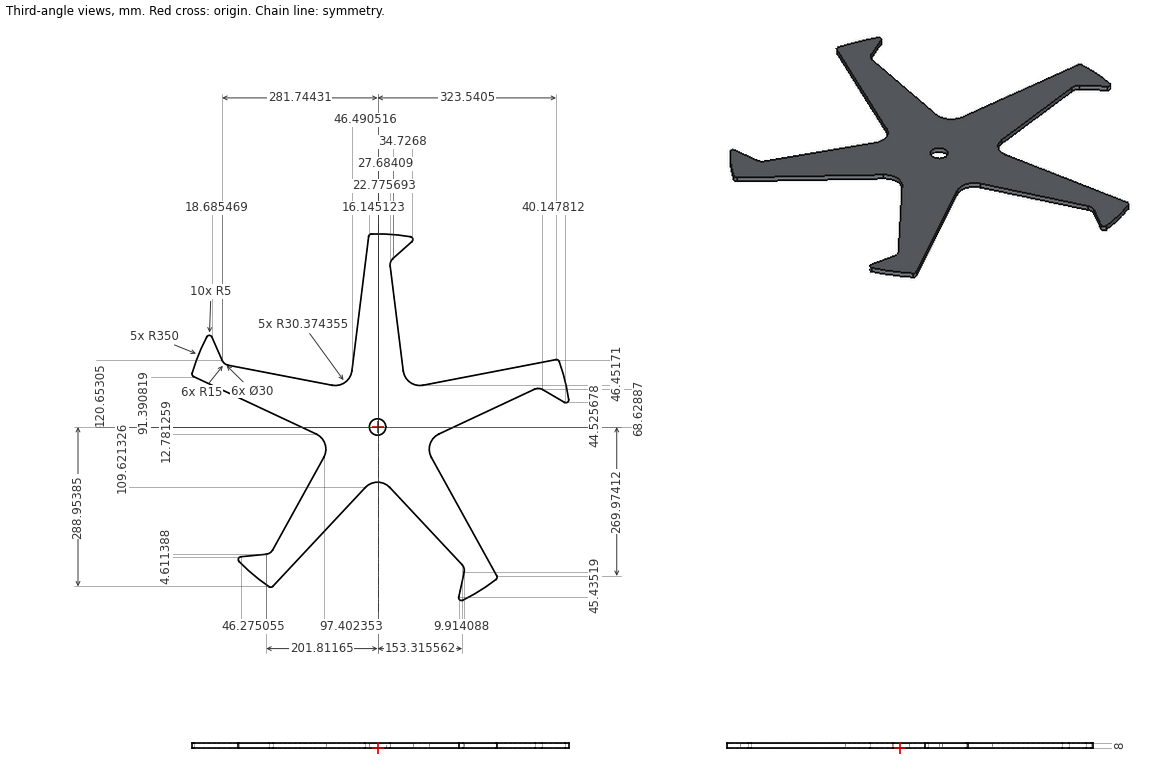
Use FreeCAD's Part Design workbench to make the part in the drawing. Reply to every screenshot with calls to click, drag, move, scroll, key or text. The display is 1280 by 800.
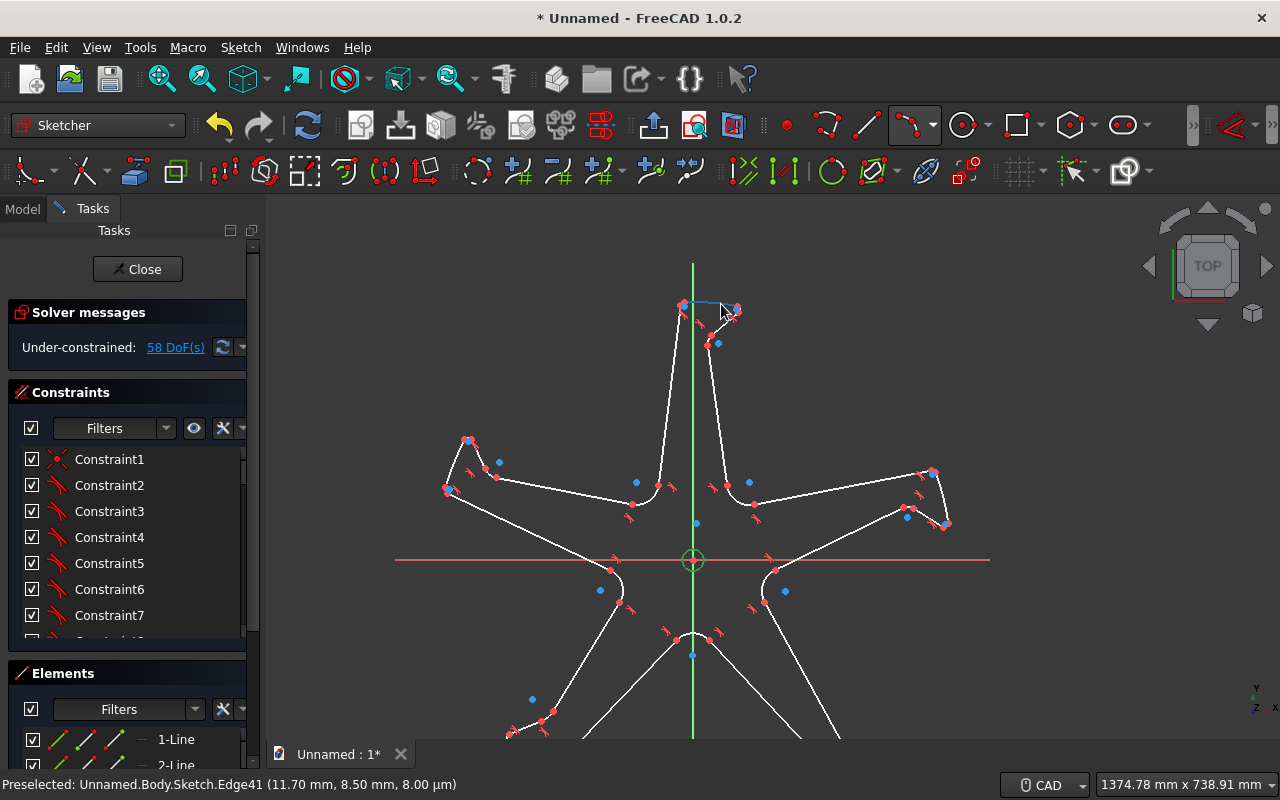
click(722, 304)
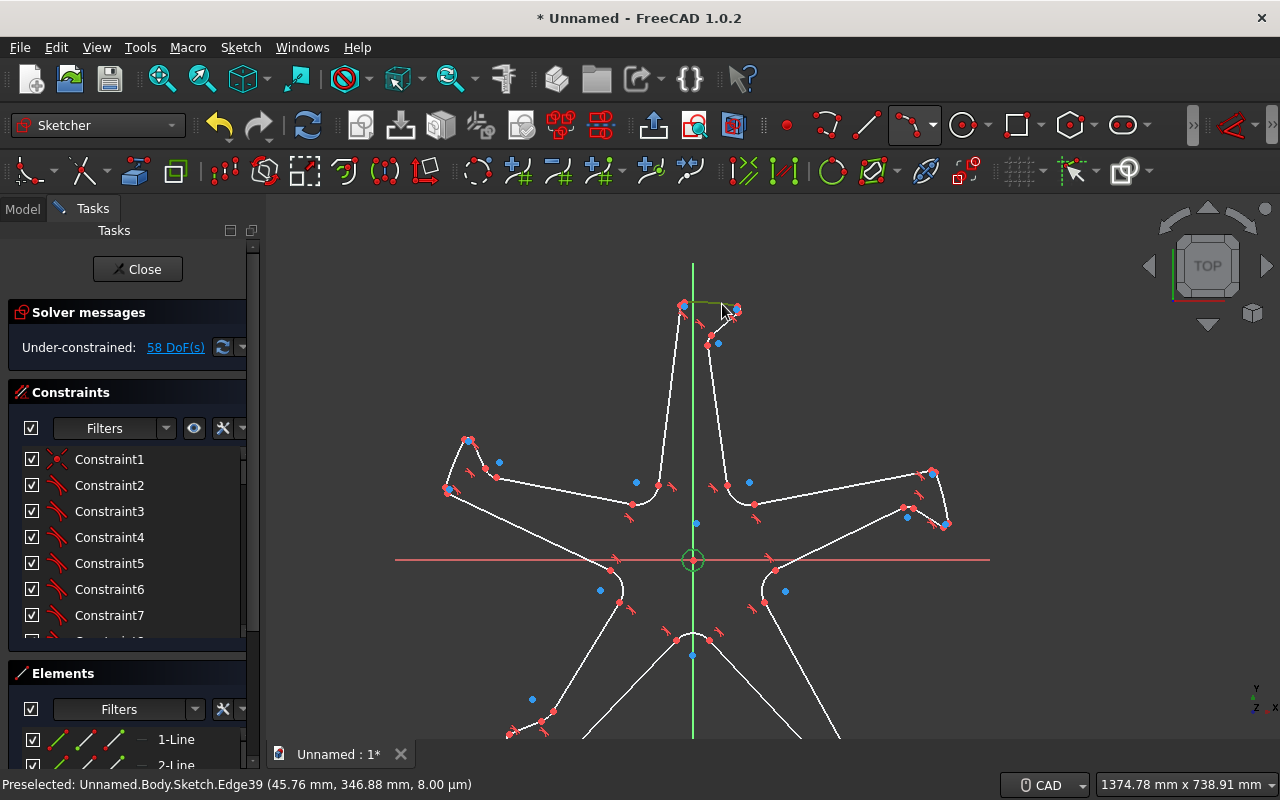
key(c)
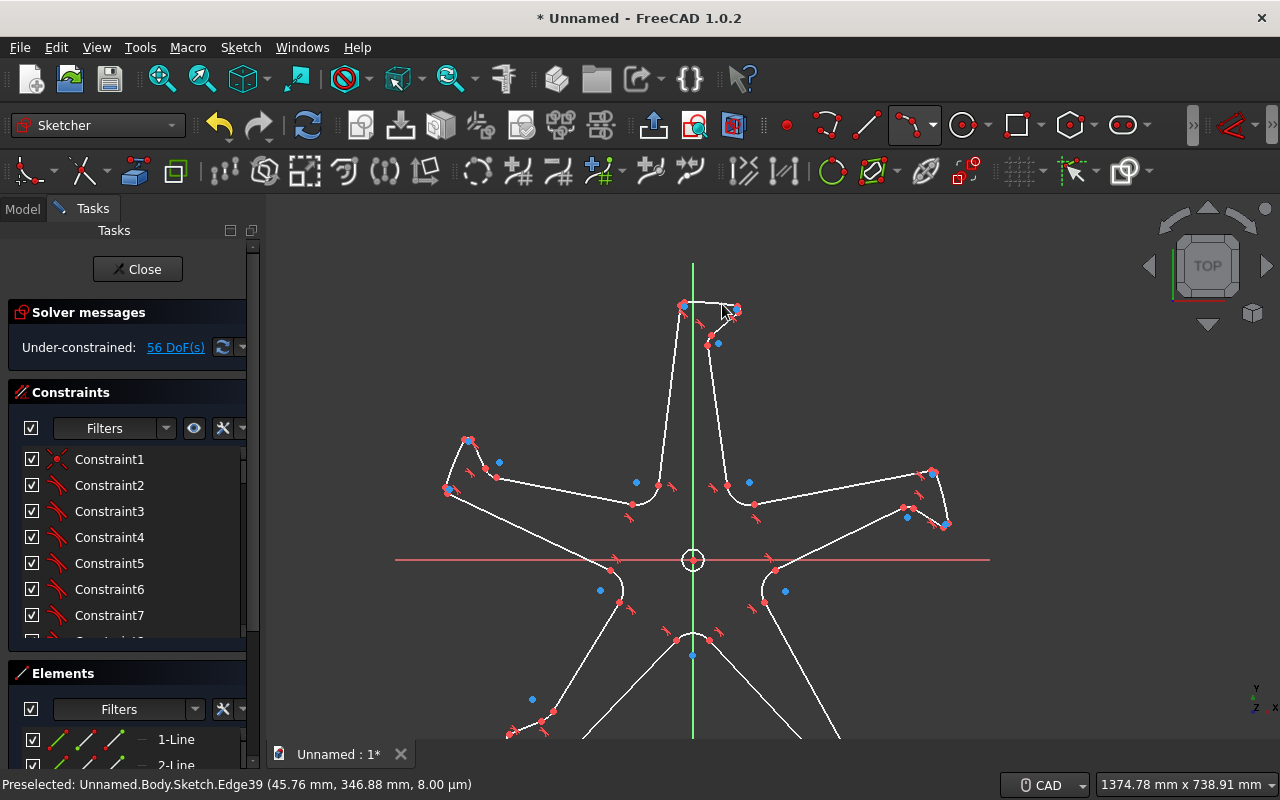
scroll(468, 438, up, 7)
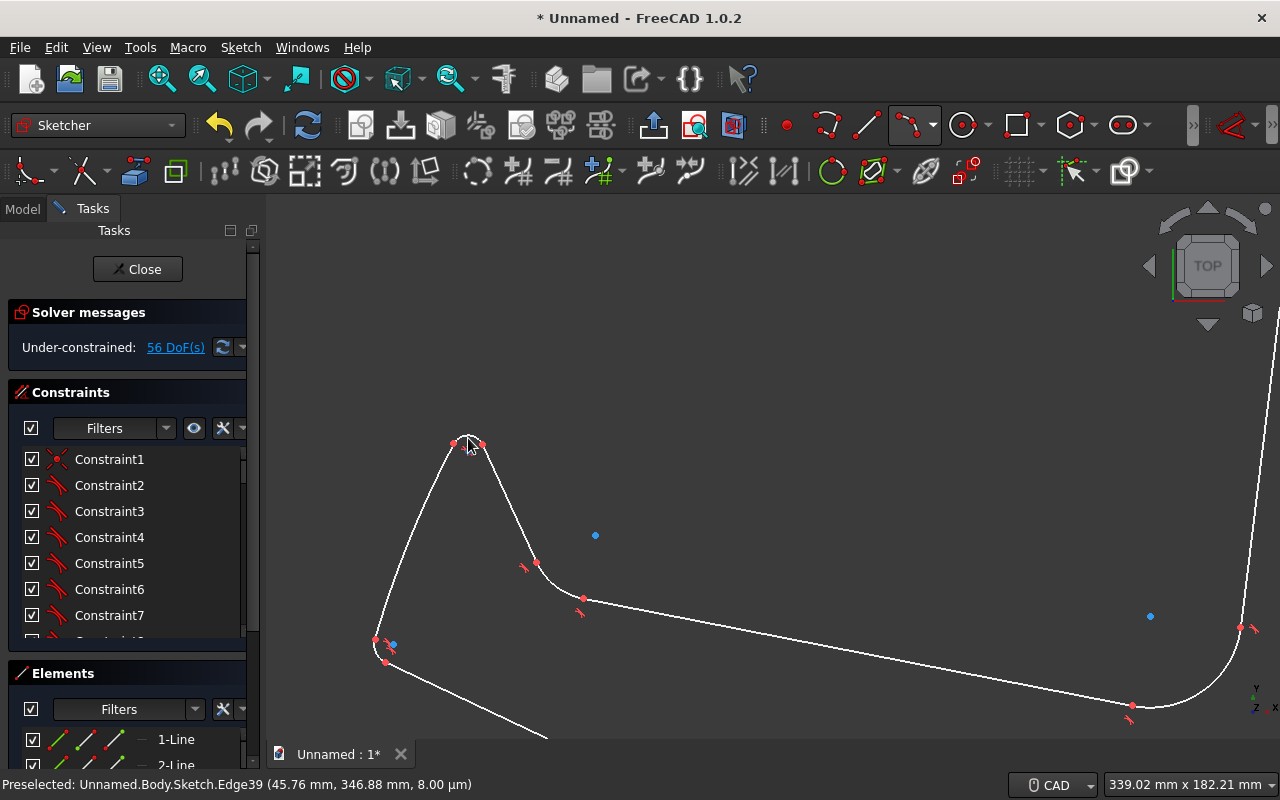
click(468, 435)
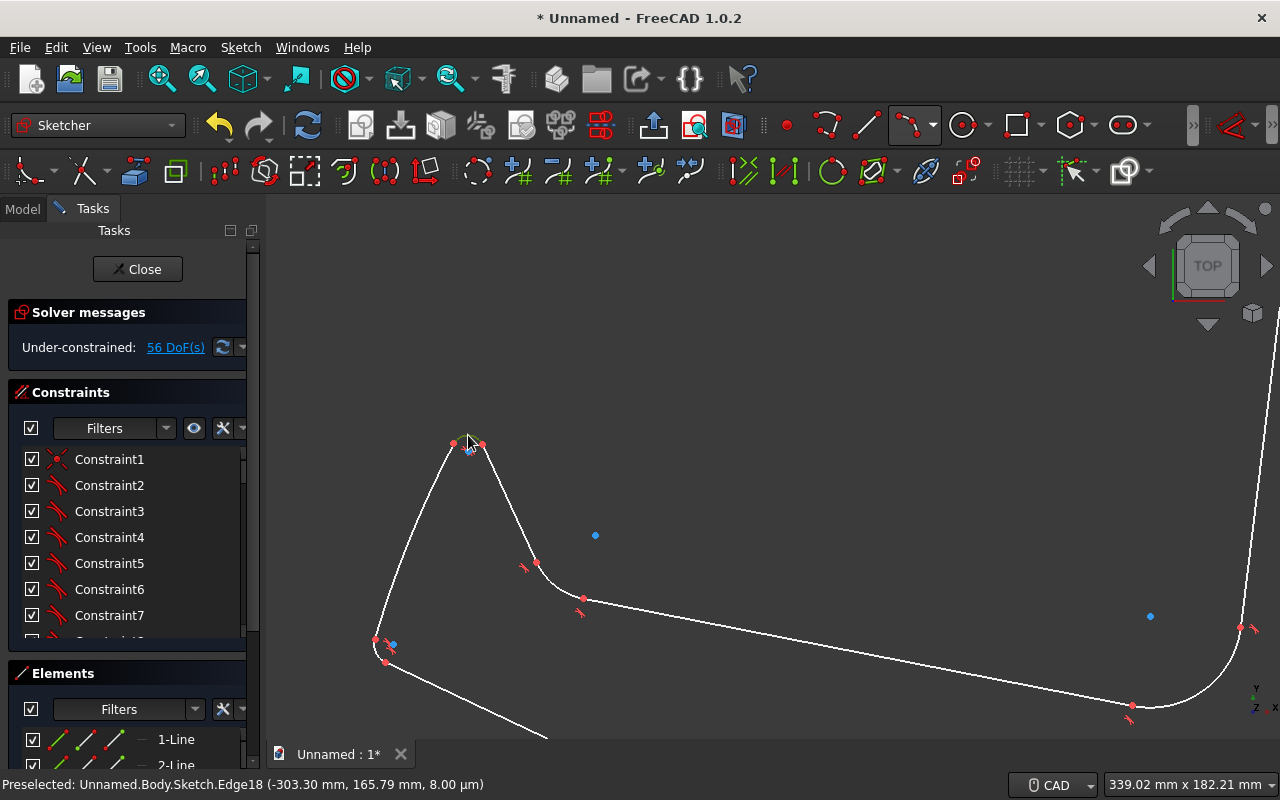
click(376, 652)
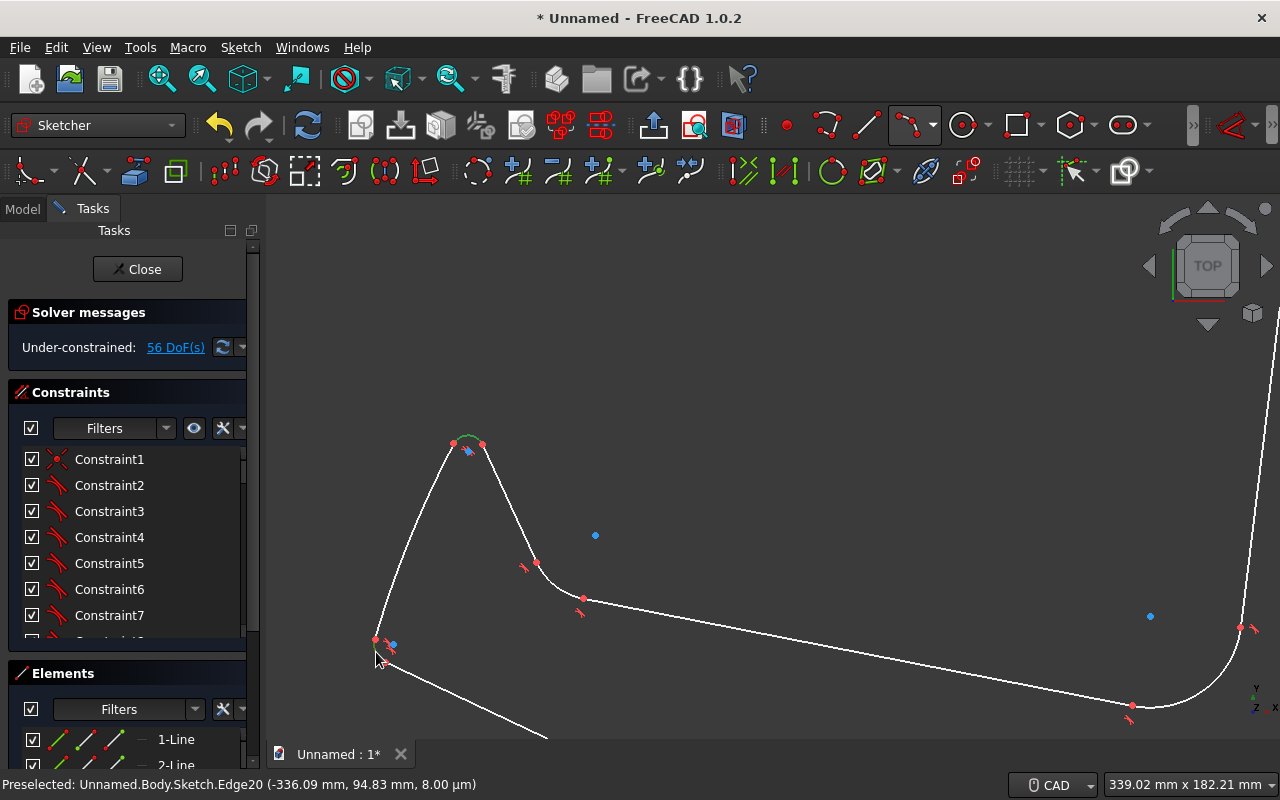
scroll(568, 385, down, 9)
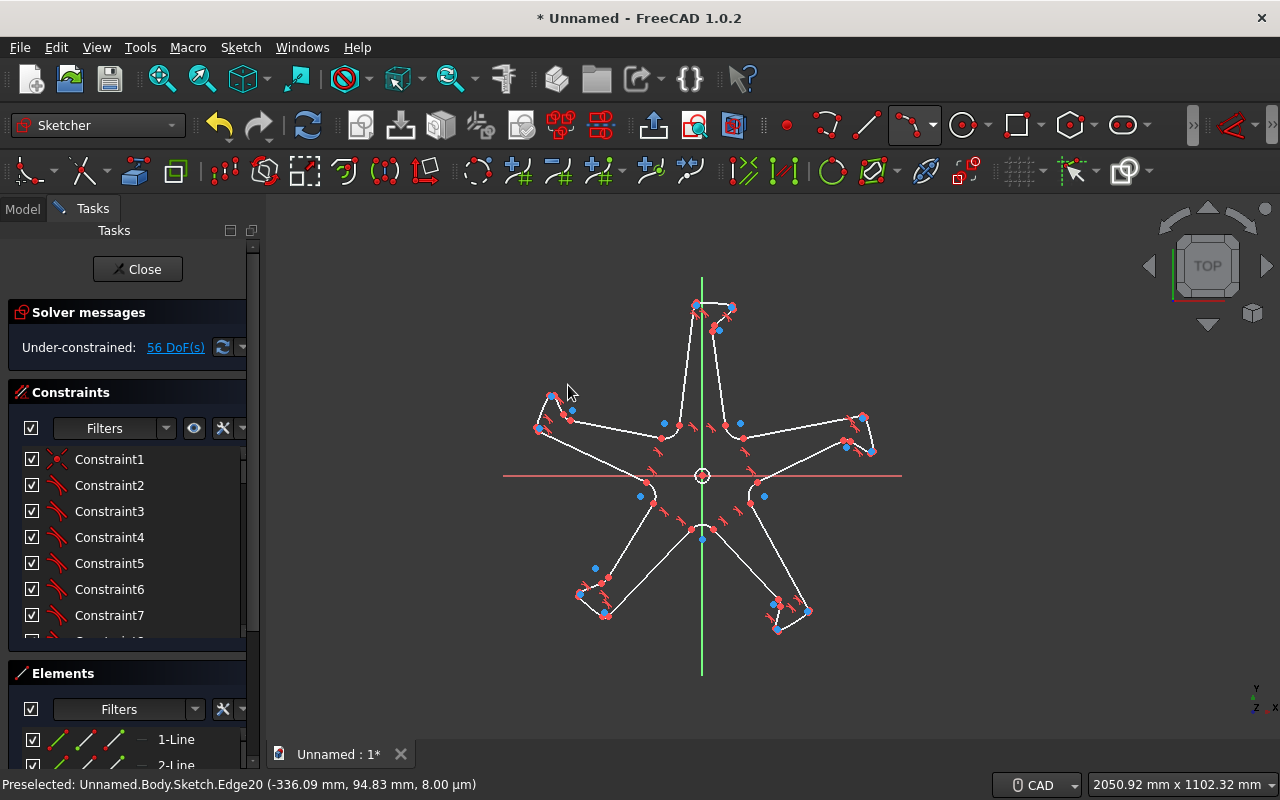
scroll(578, 593, up, 11)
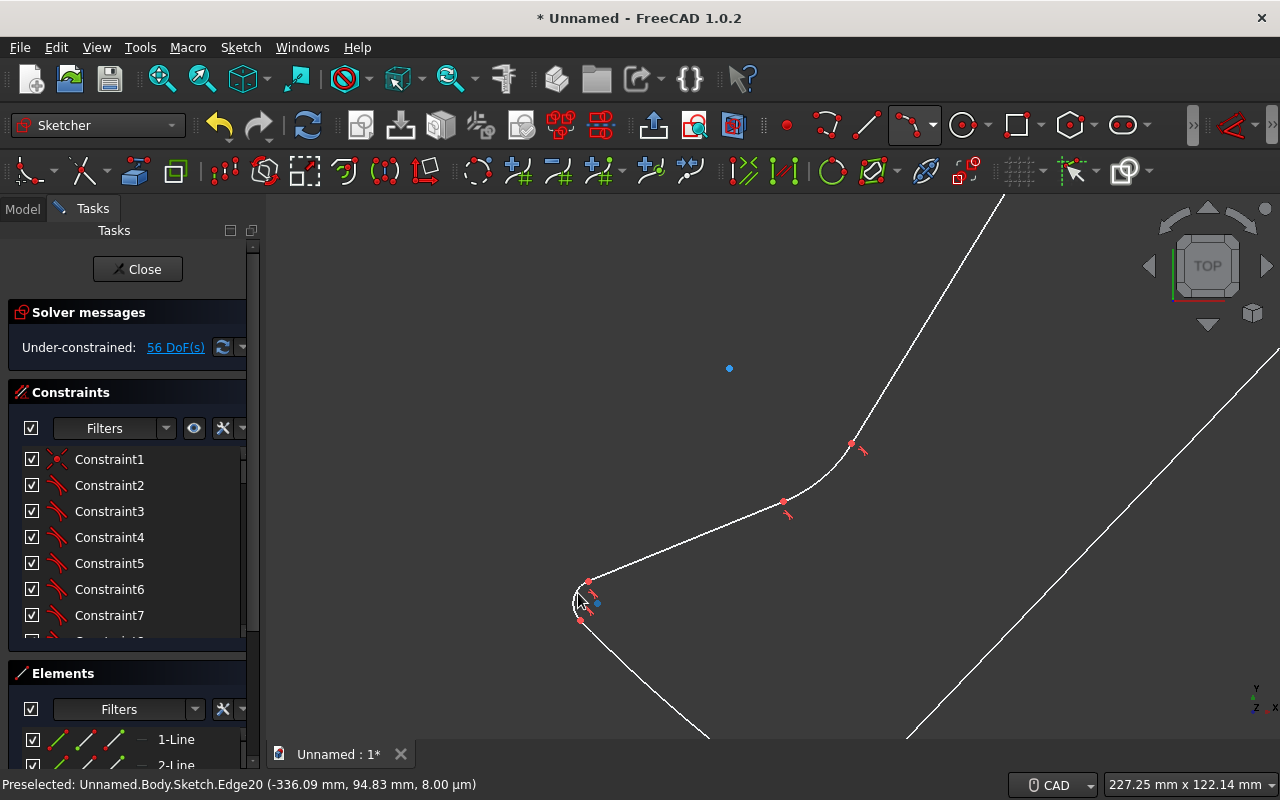
click(578, 590)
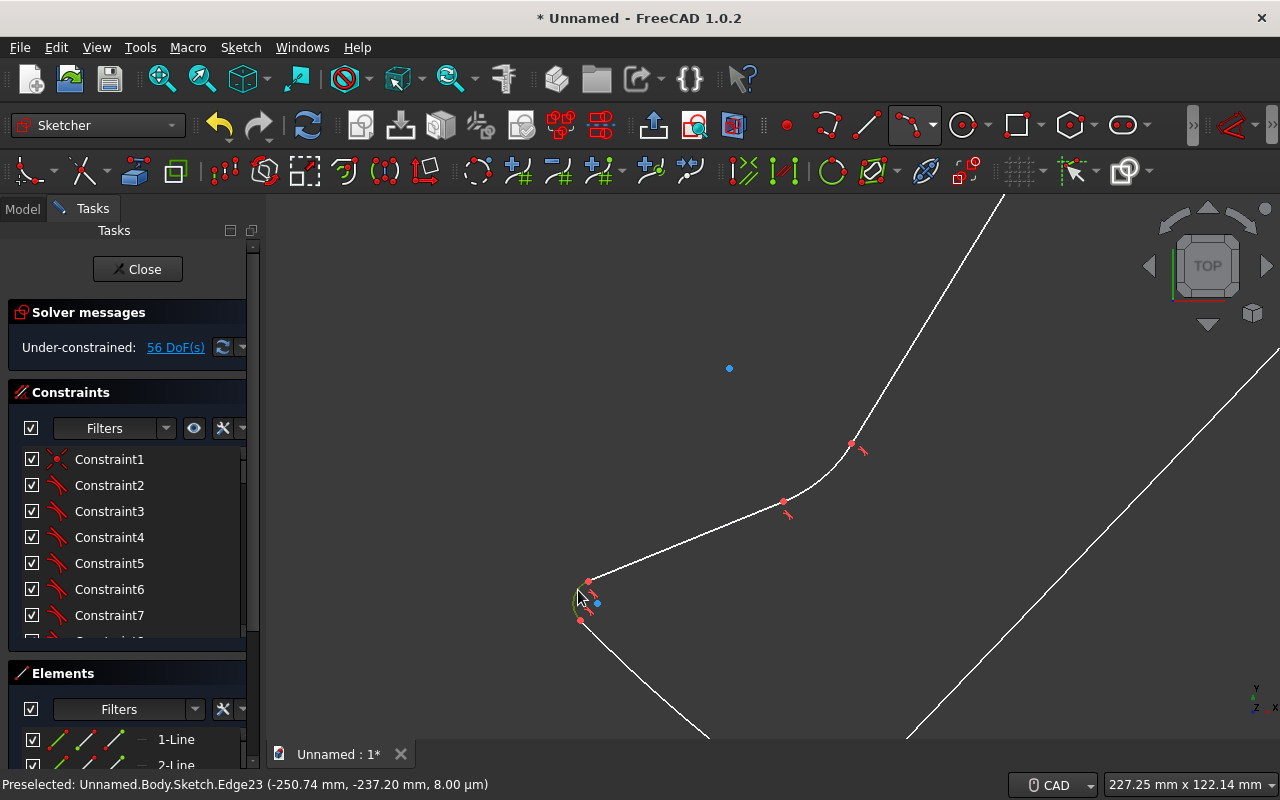
scroll(578, 593, down, 11)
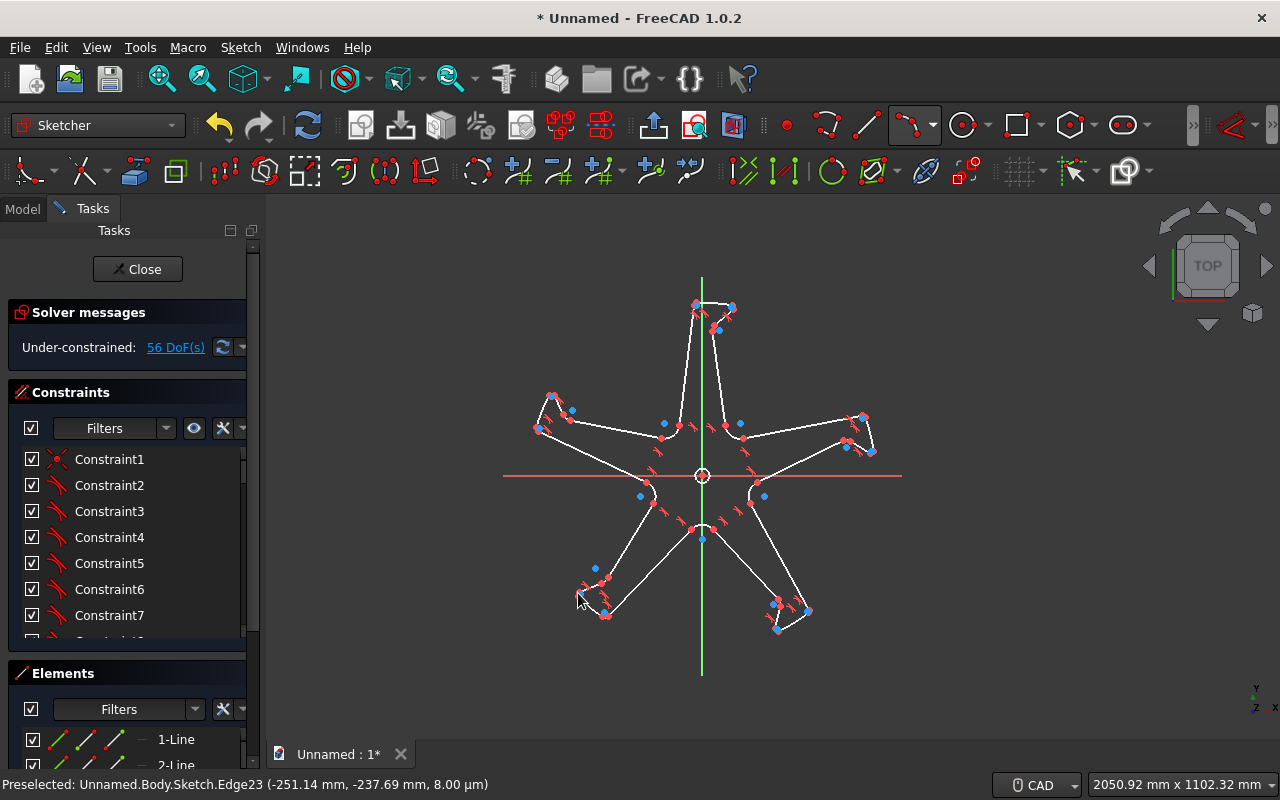
scroll(604, 618, up, 10)